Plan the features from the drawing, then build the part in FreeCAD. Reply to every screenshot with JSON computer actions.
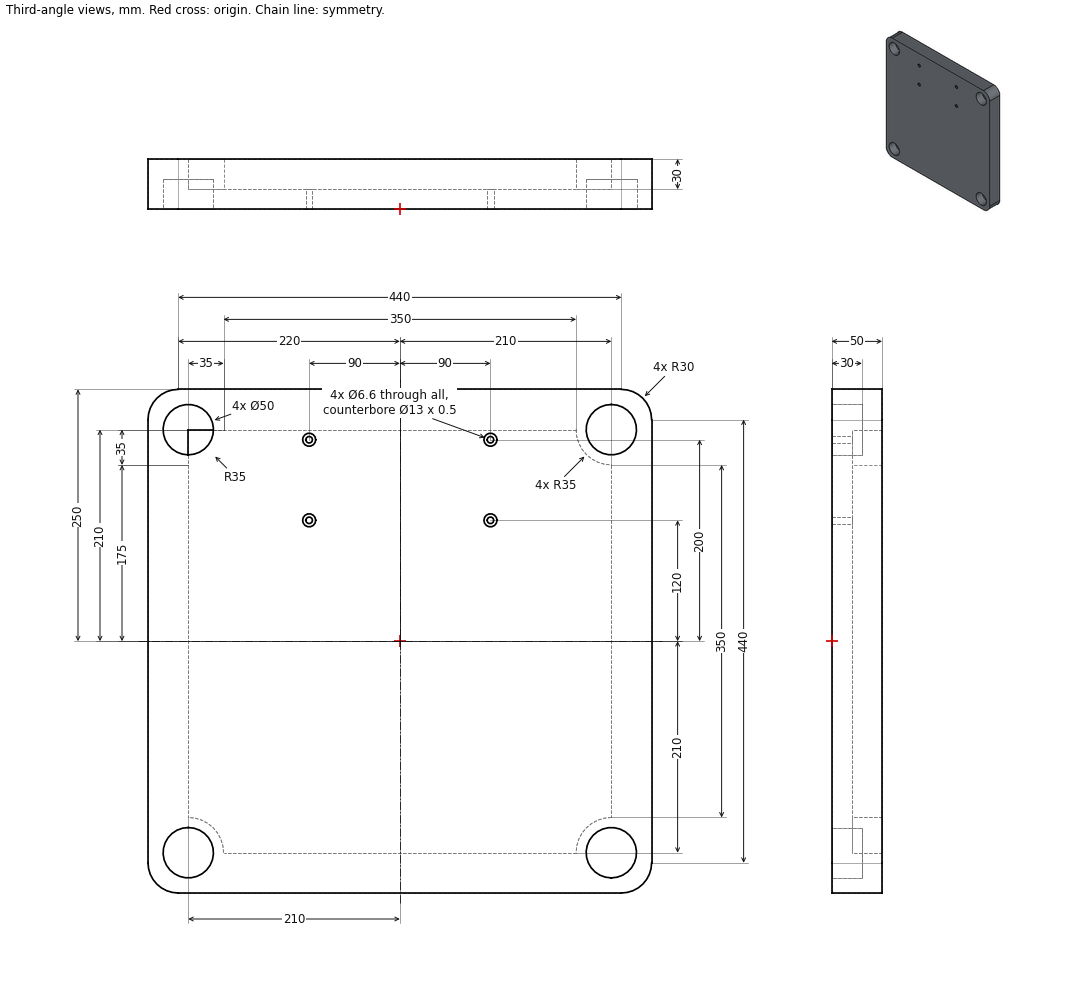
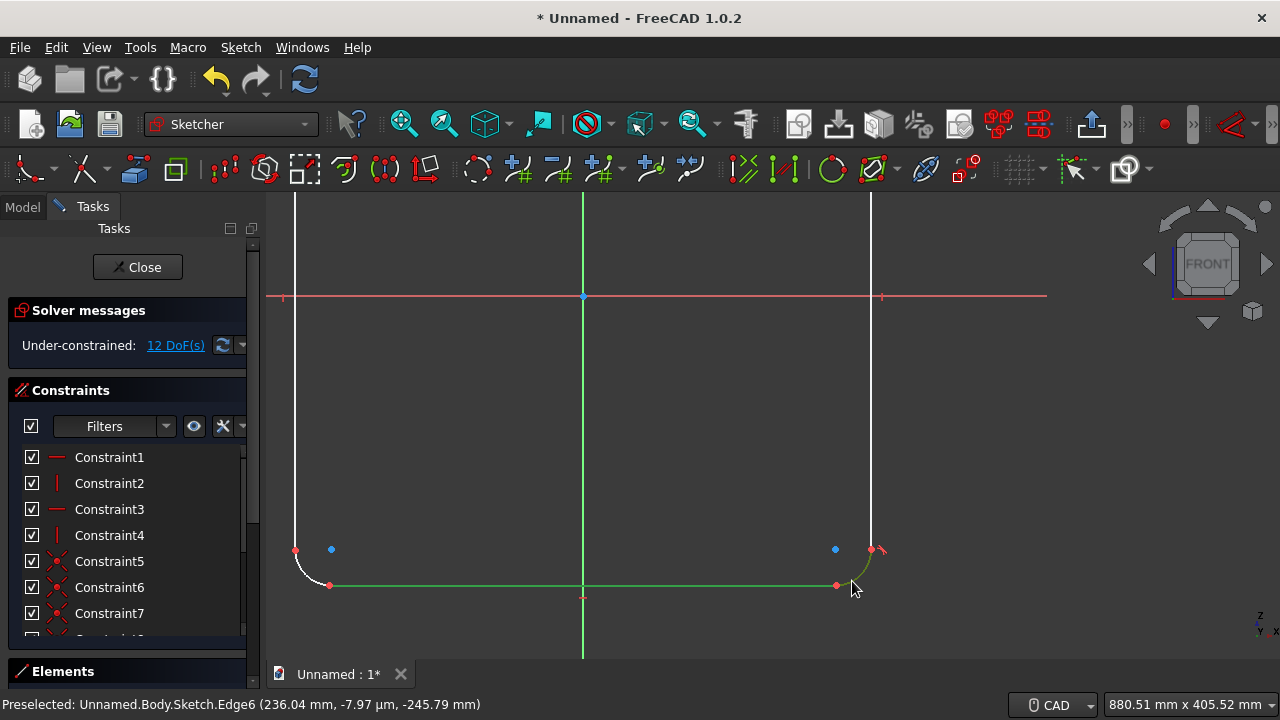
{"action": "key", "text": "t"}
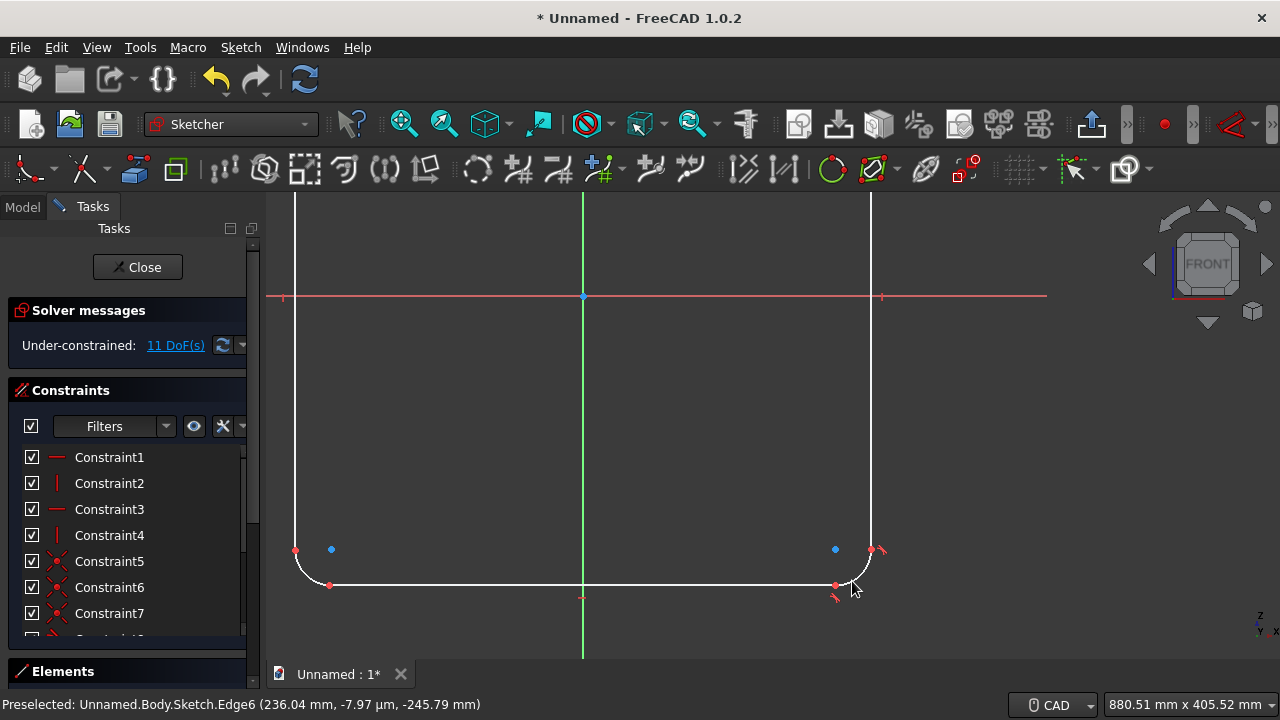
{"action": "left_click", "coordinate": [684, 585]}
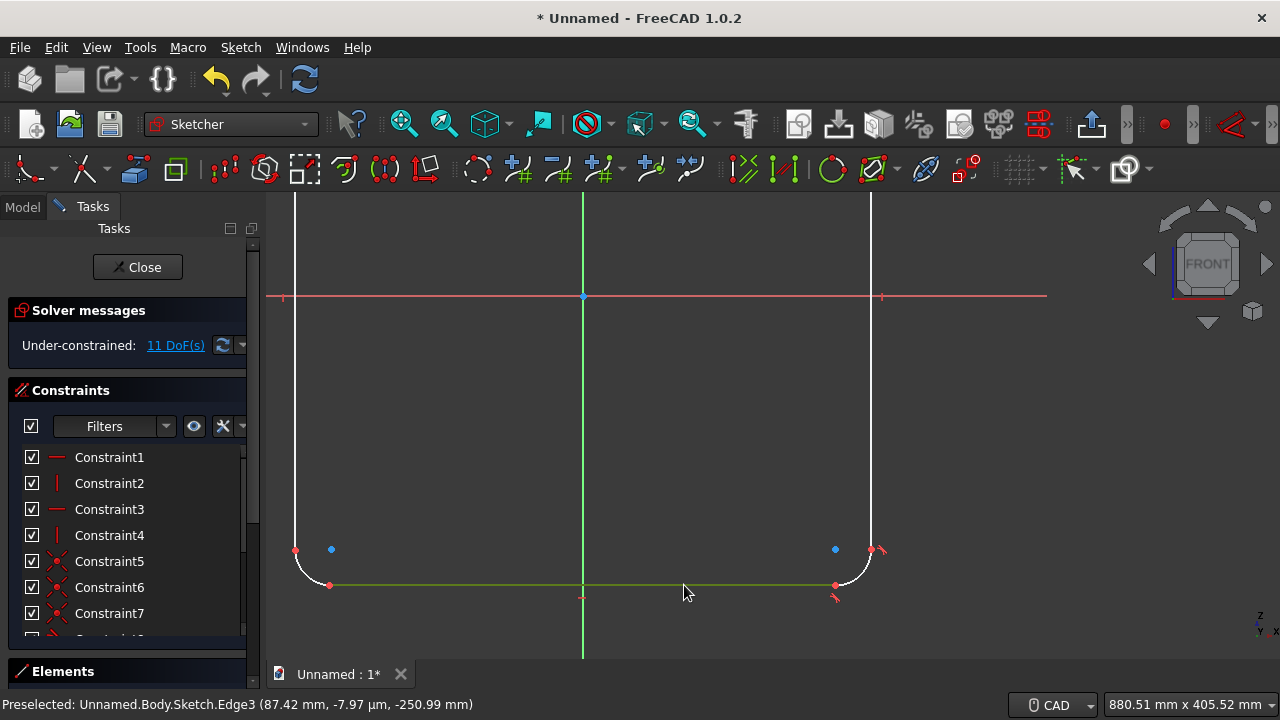
{"action": "left_click", "coordinate": [300, 566]}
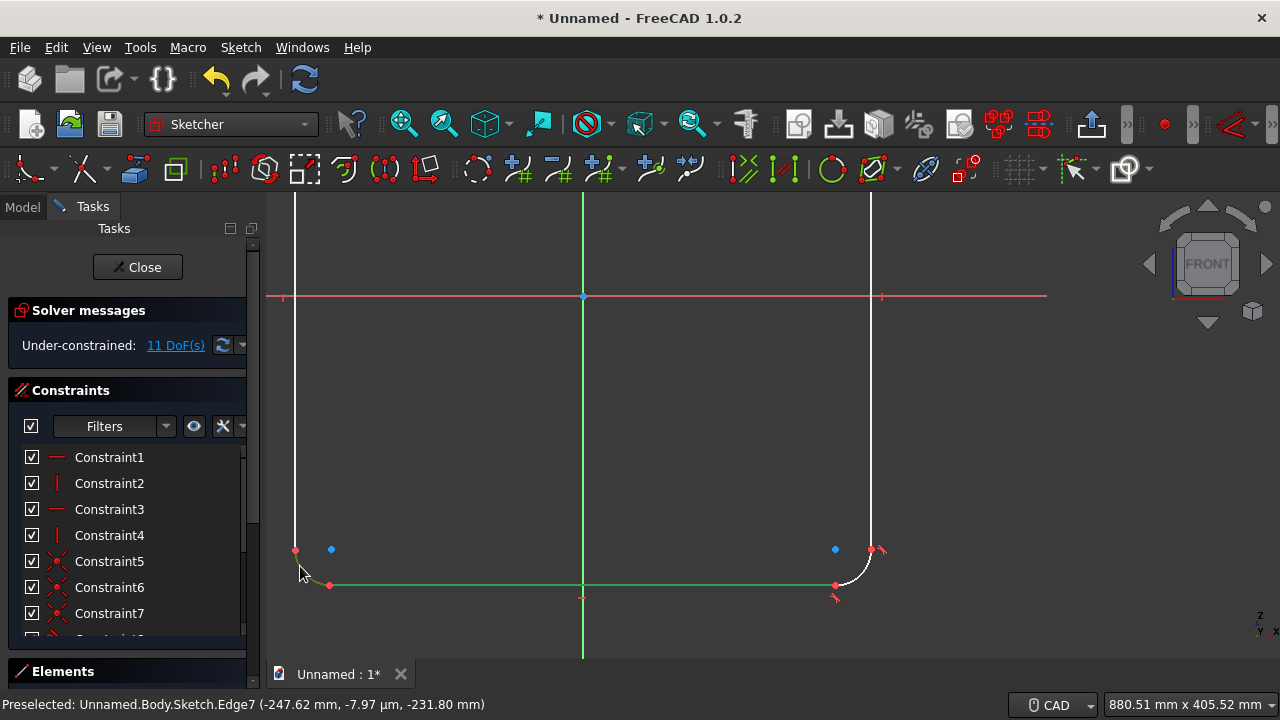
{"action": "key", "text": "t"}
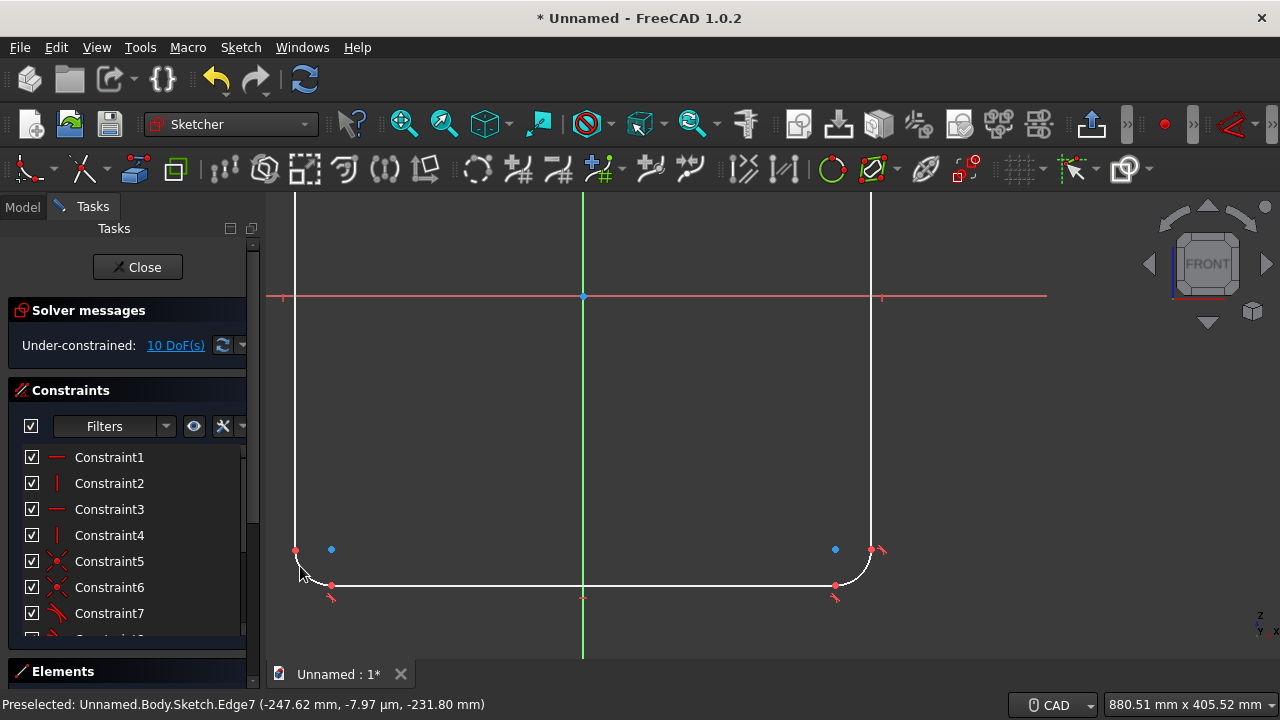
{"action": "left_click", "coordinate": [295, 399]}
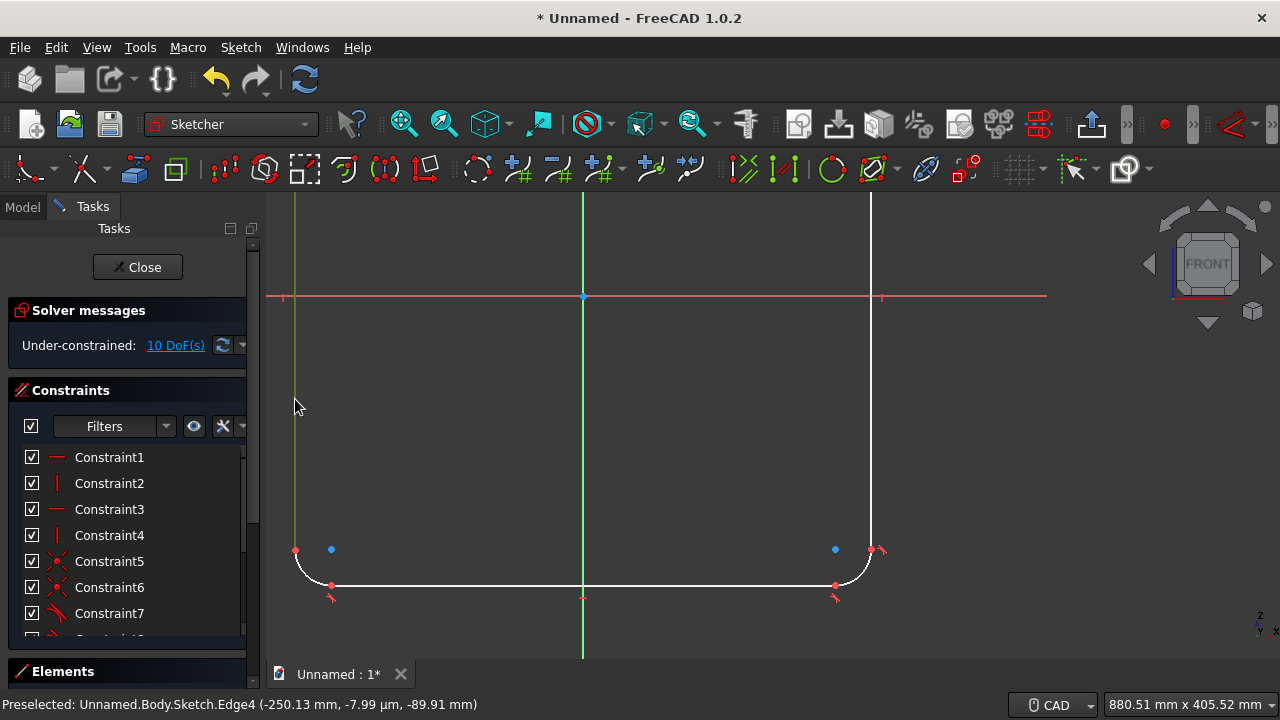
{"action": "left_click", "coordinate": [300, 567]}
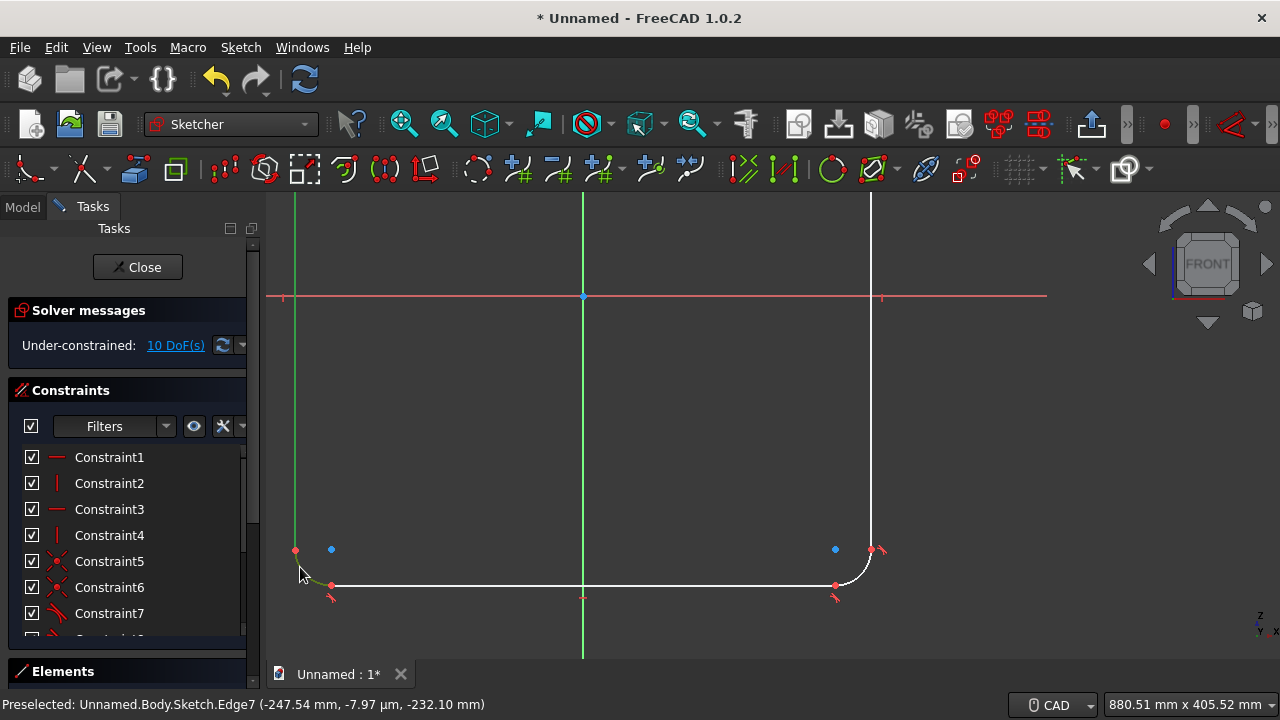
{"action": "key", "text": "t"}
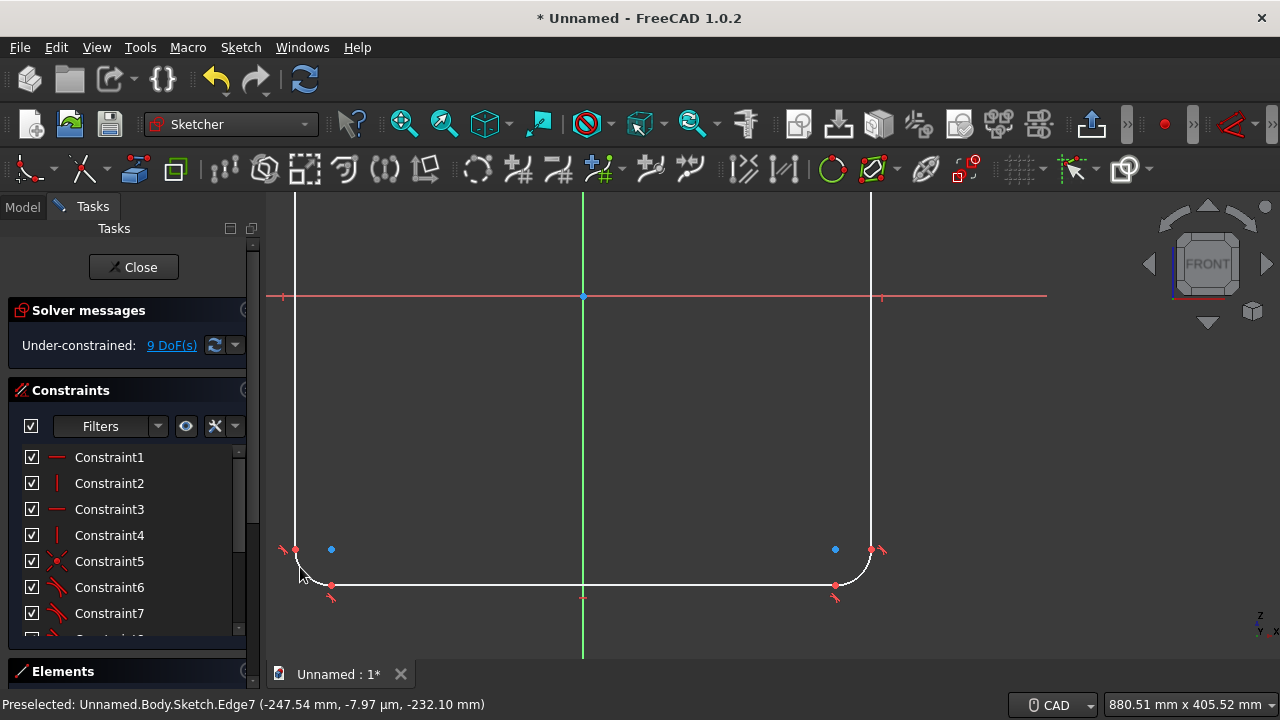
{"action": "left_click", "coordinate": [295, 398]}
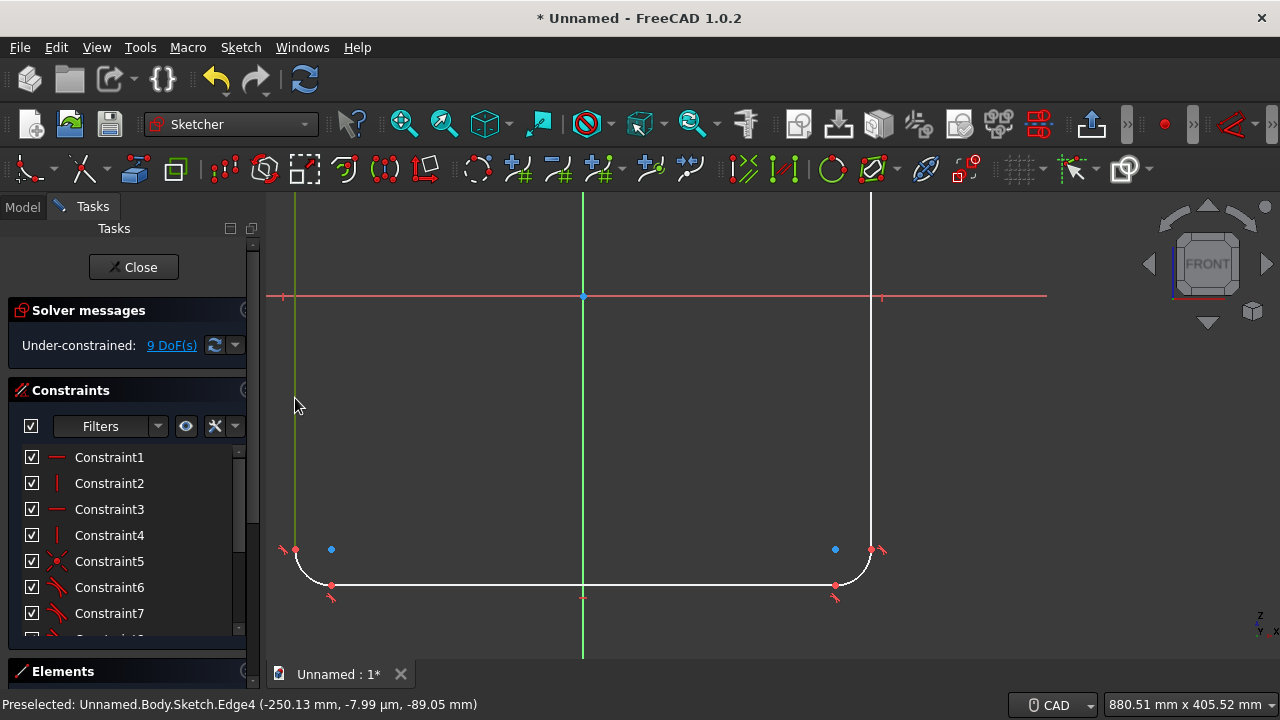
{"action": "scroll", "coordinate": [852, 582], "scroll_direction": "down", "scroll_amount": 3}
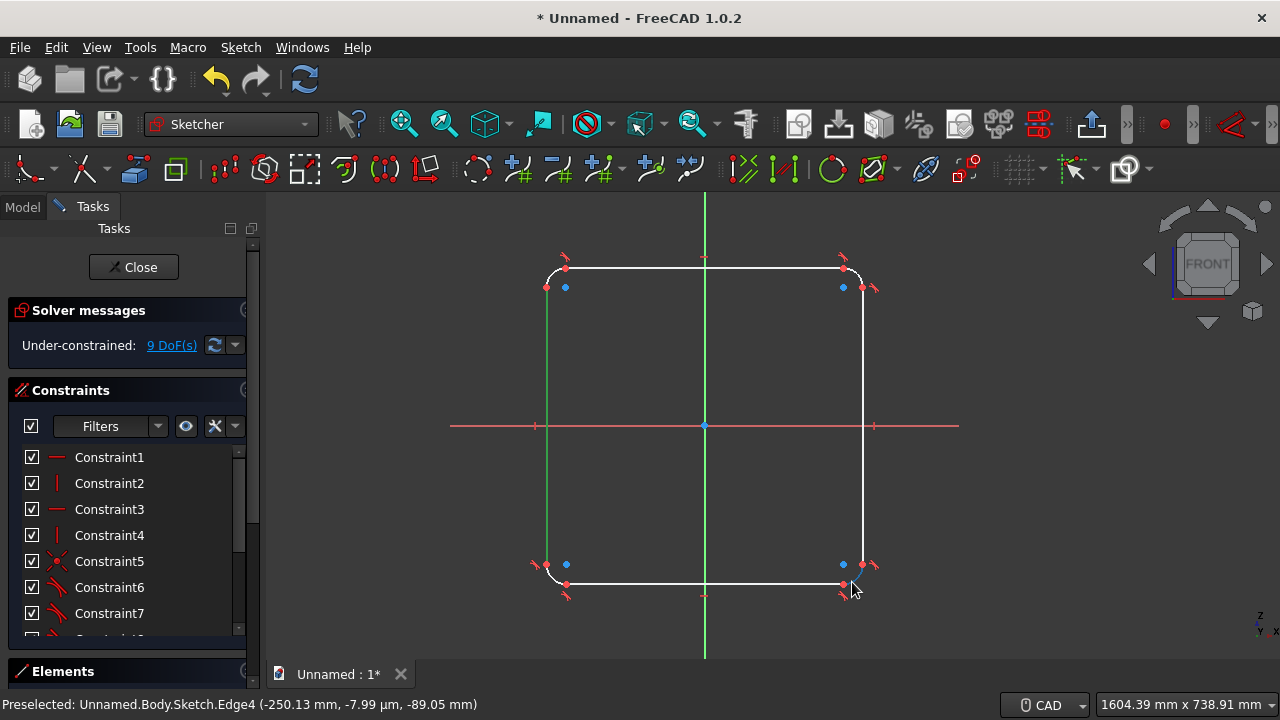
{"action": "scroll", "coordinate": [557, 270], "scroll_direction": "up", "scroll_amount": 3}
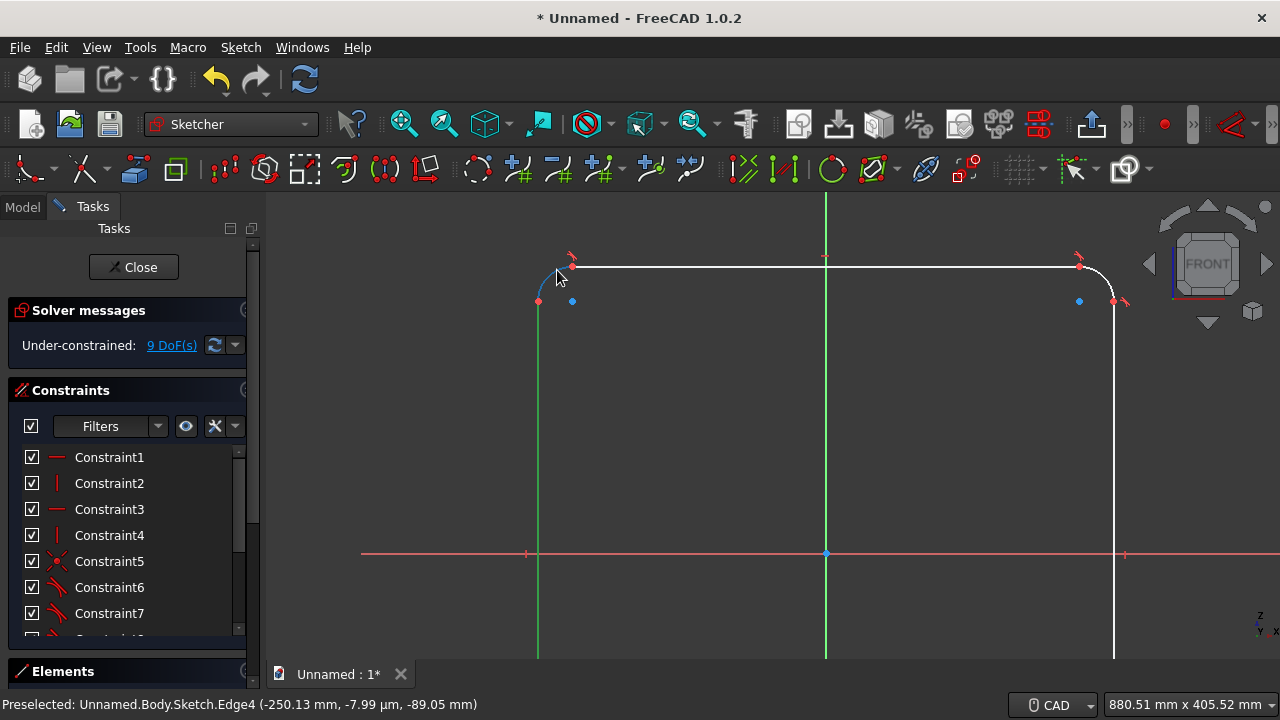
{"action": "left_click", "coordinate": [557, 271]}